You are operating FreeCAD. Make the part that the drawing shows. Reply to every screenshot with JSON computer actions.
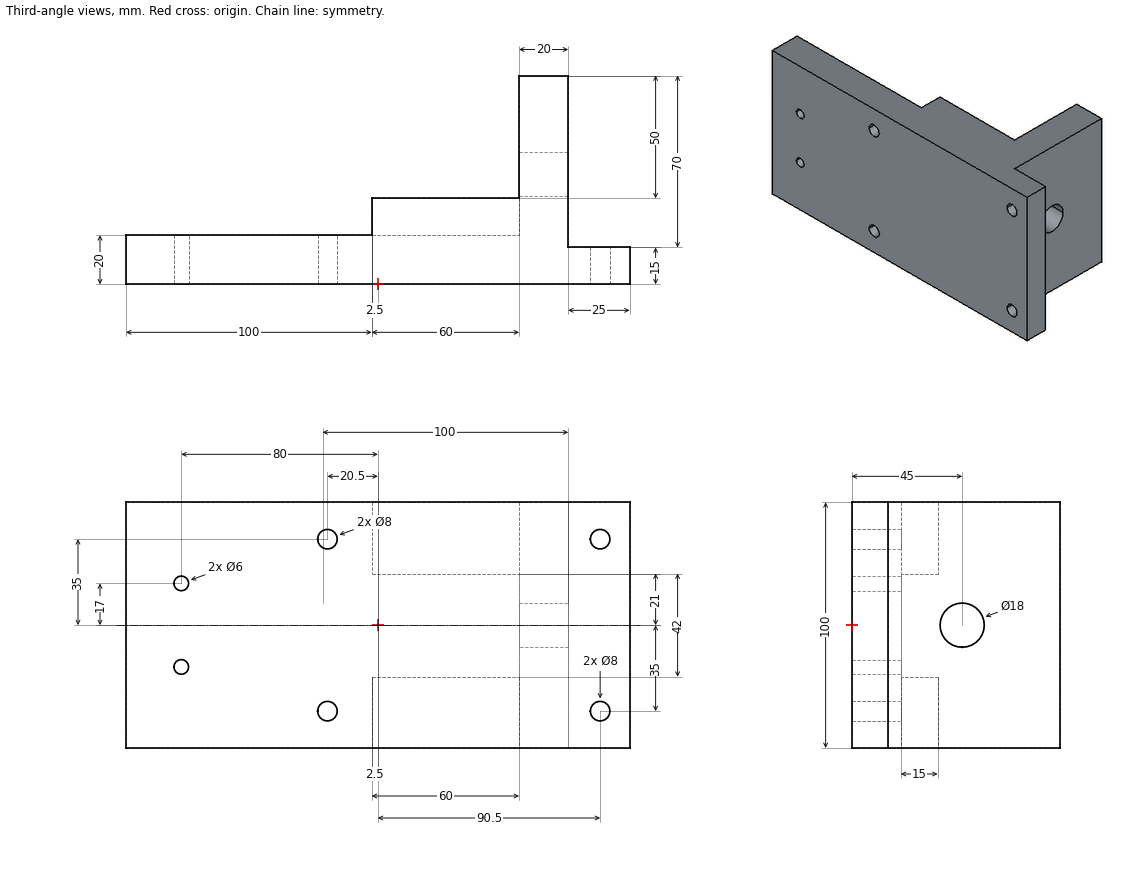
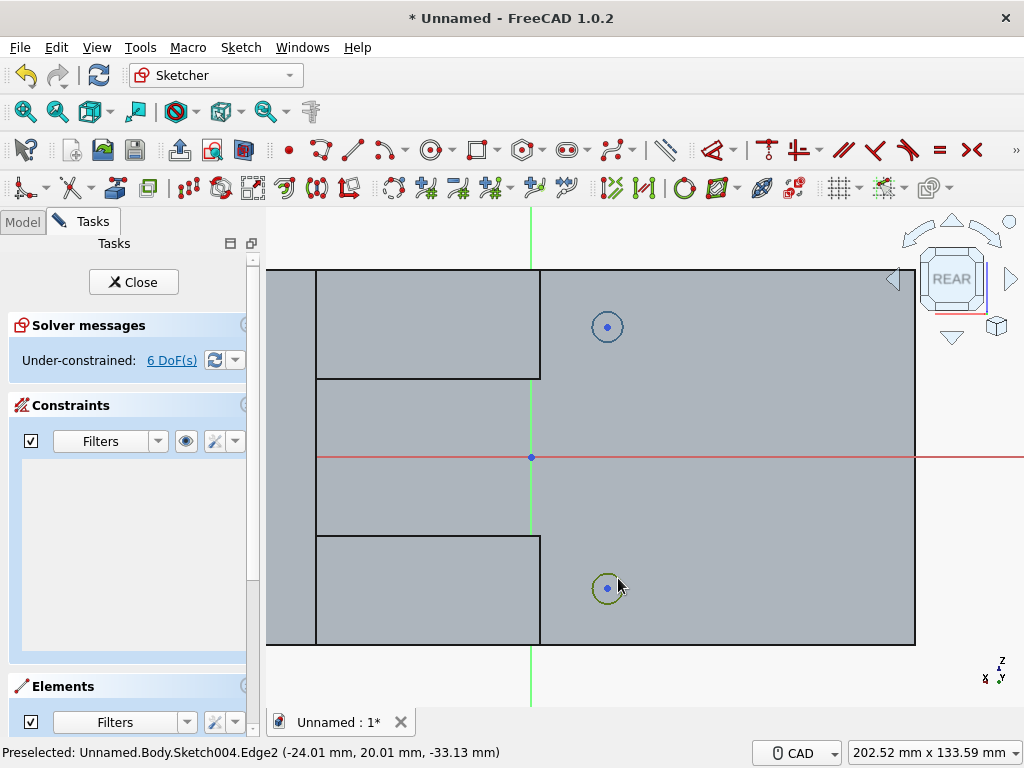
{"action": "left_click", "coordinate": [940, 150]}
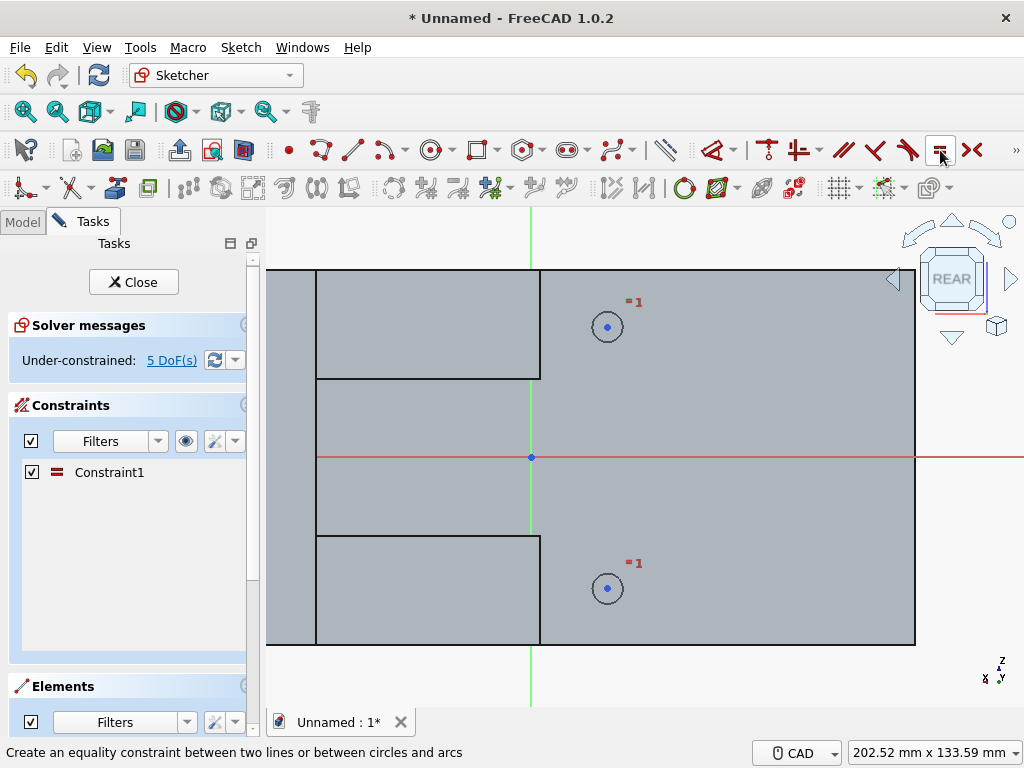
{"action": "left_click", "coordinate": [608, 327]}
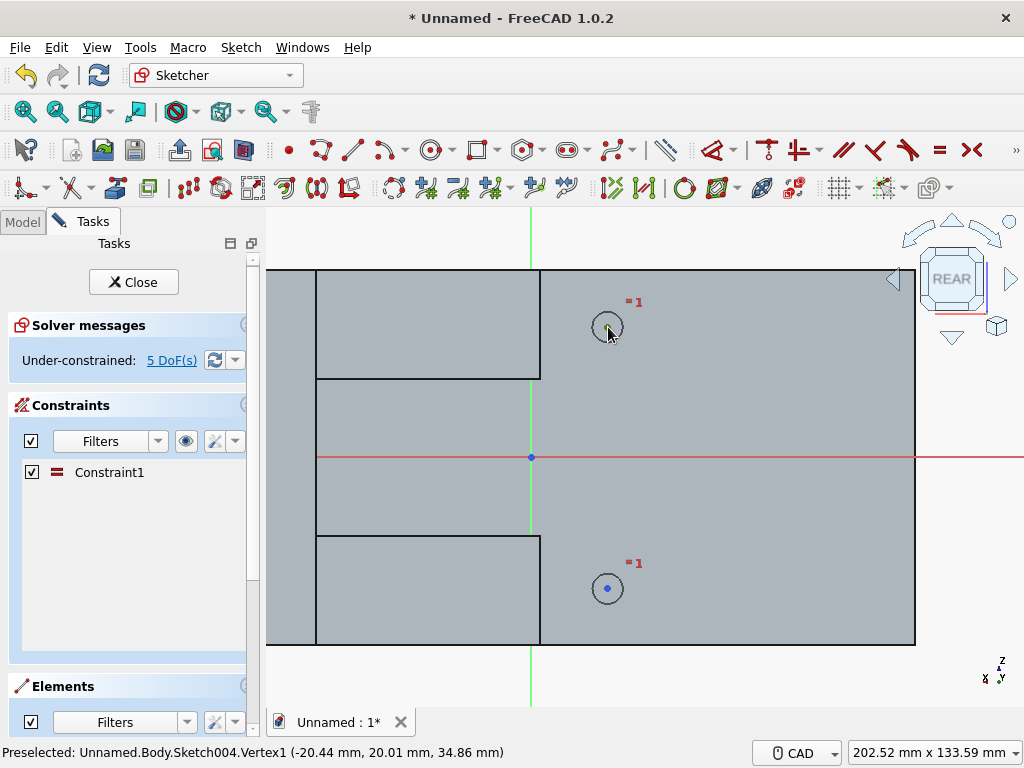
{"action": "left_click", "coordinate": [608, 589]}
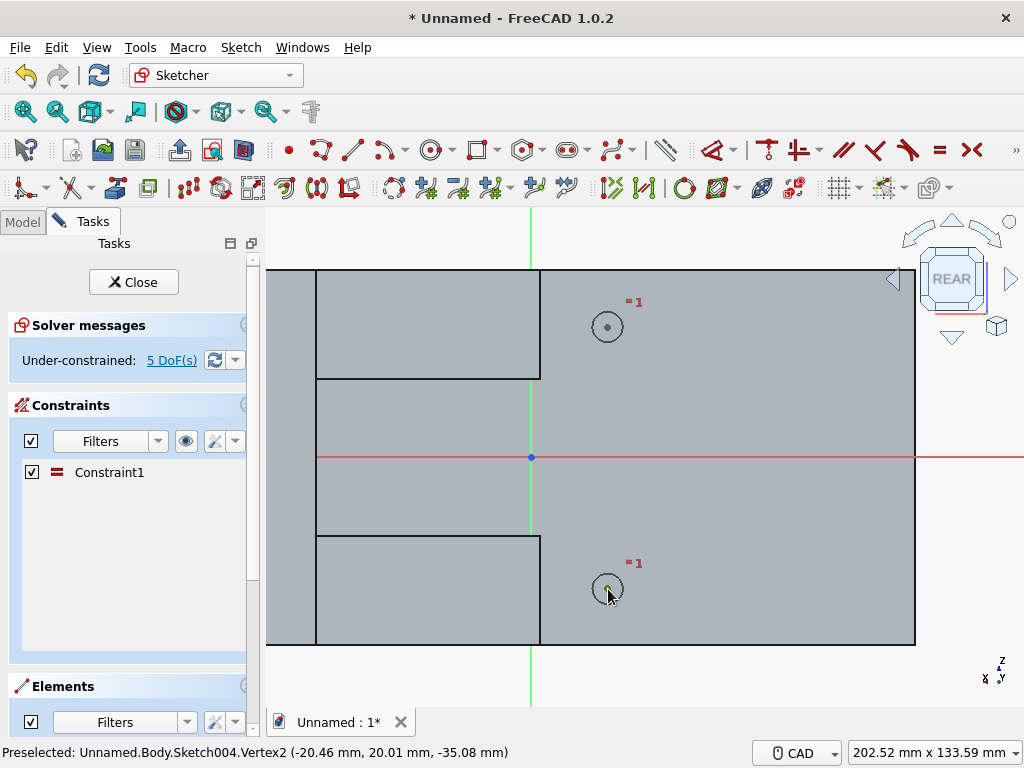
{"action": "left_click", "coordinate": [334, 457]}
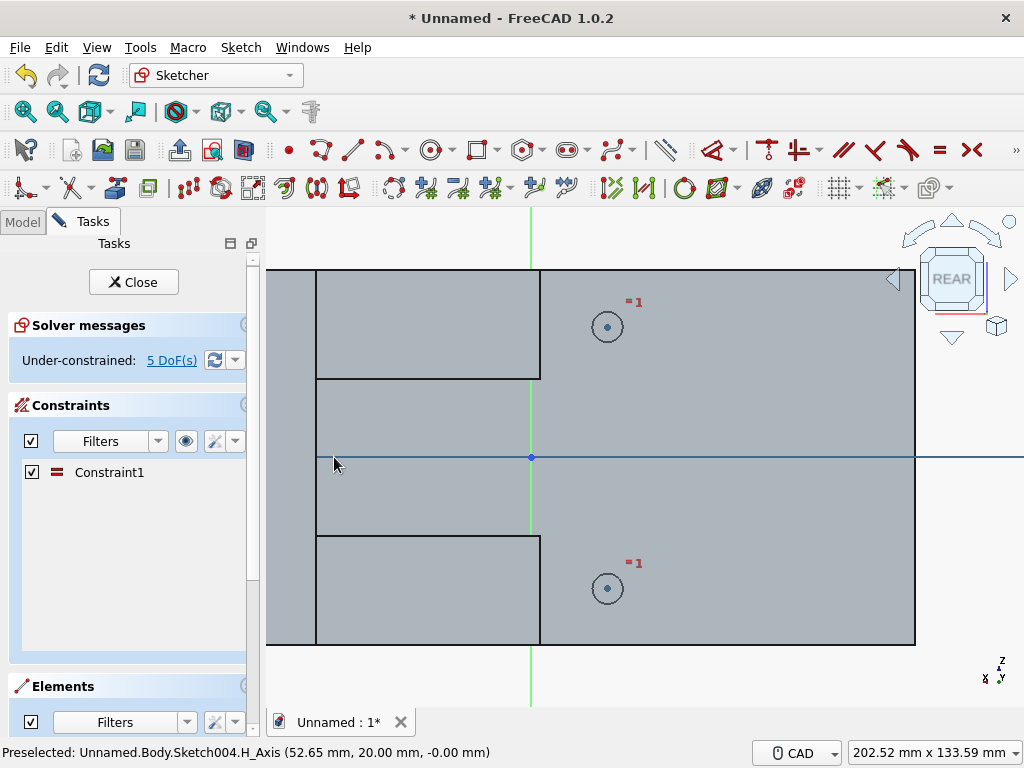
{"action": "left_click", "coordinate": [972, 150]}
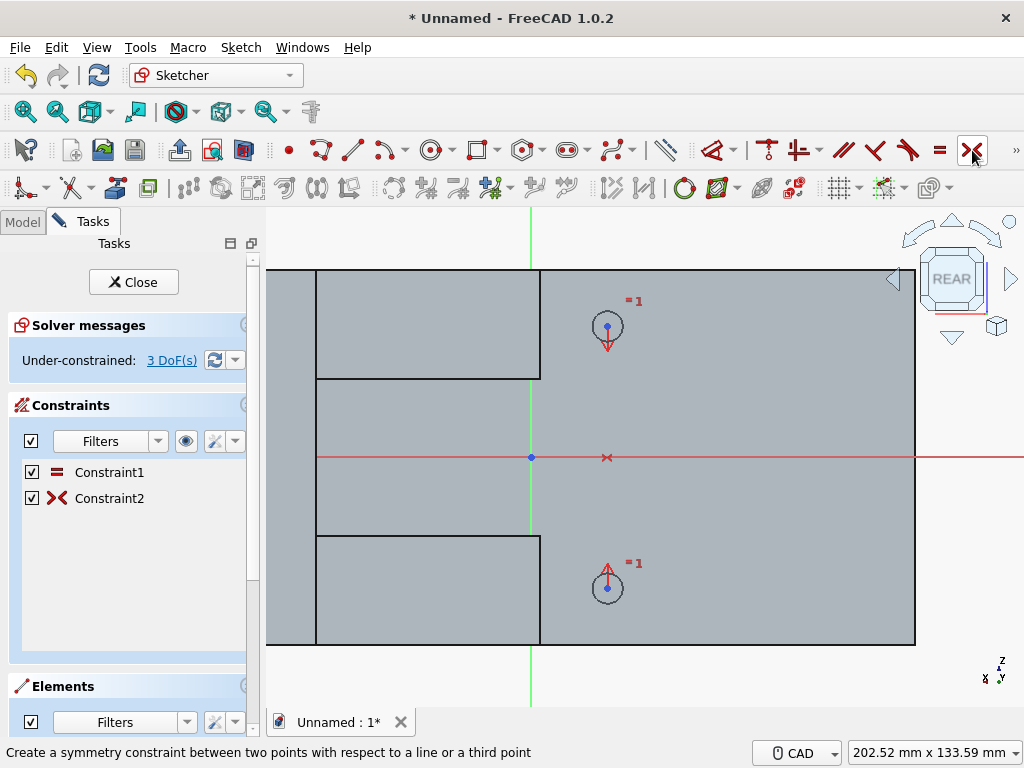
{"action": "left_click", "coordinate": [712, 150]}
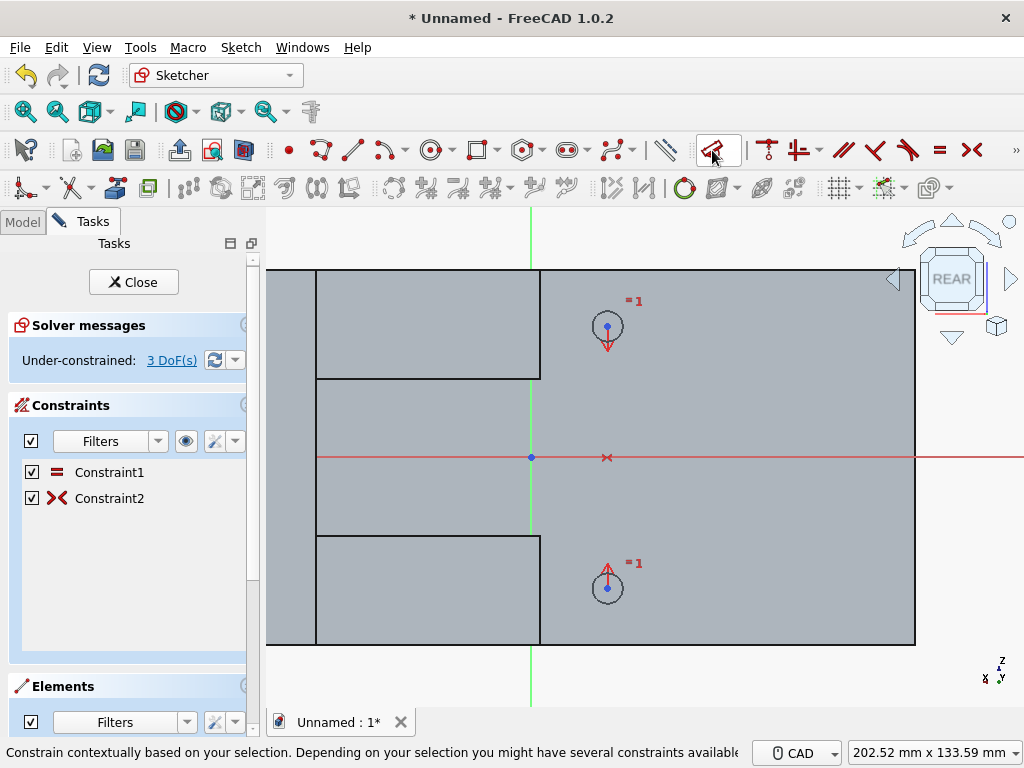
{"action": "scroll", "coordinate": [618, 316], "scroll_direction": "up", "scroll_amount": 2}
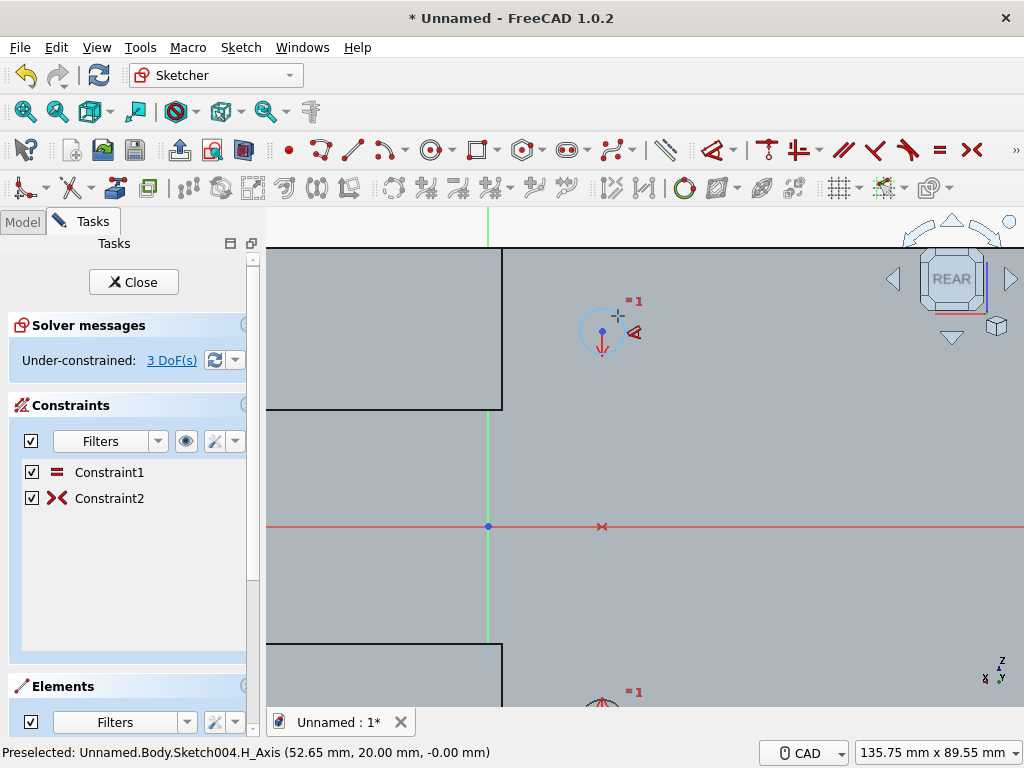
{"action": "left_click", "coordinate": [618, 315]}
{"action": "left_click", "coordinate": [640, 292]}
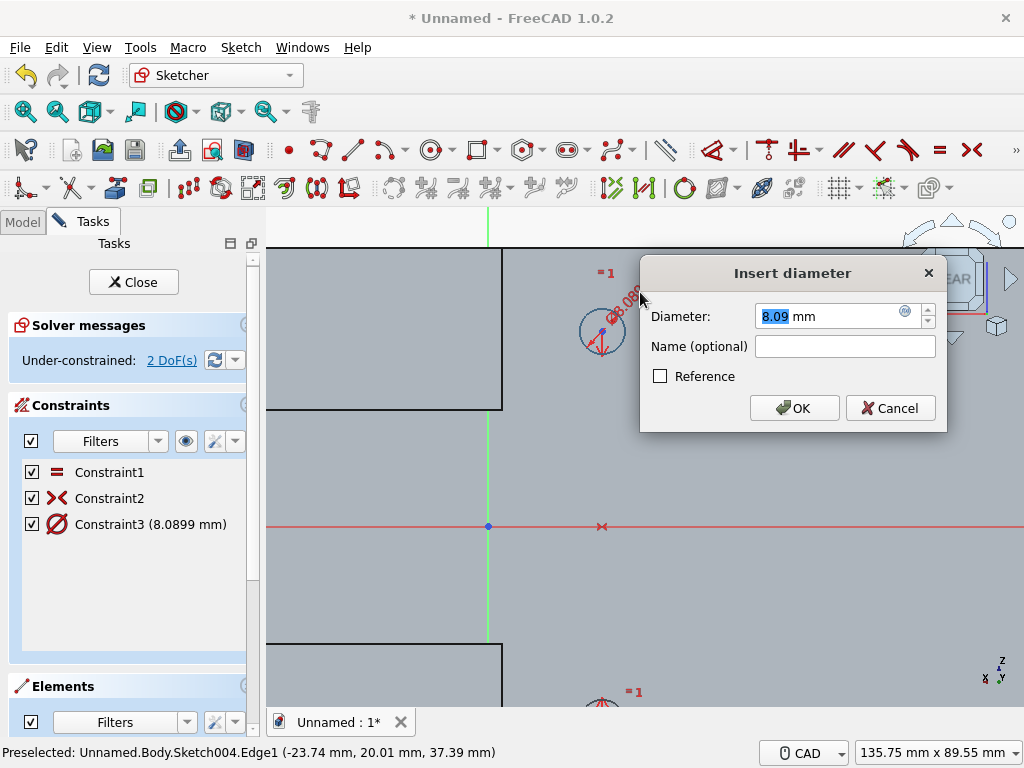
{"action": "type", "text": "8"}
{"action": "key", "text": "Return"}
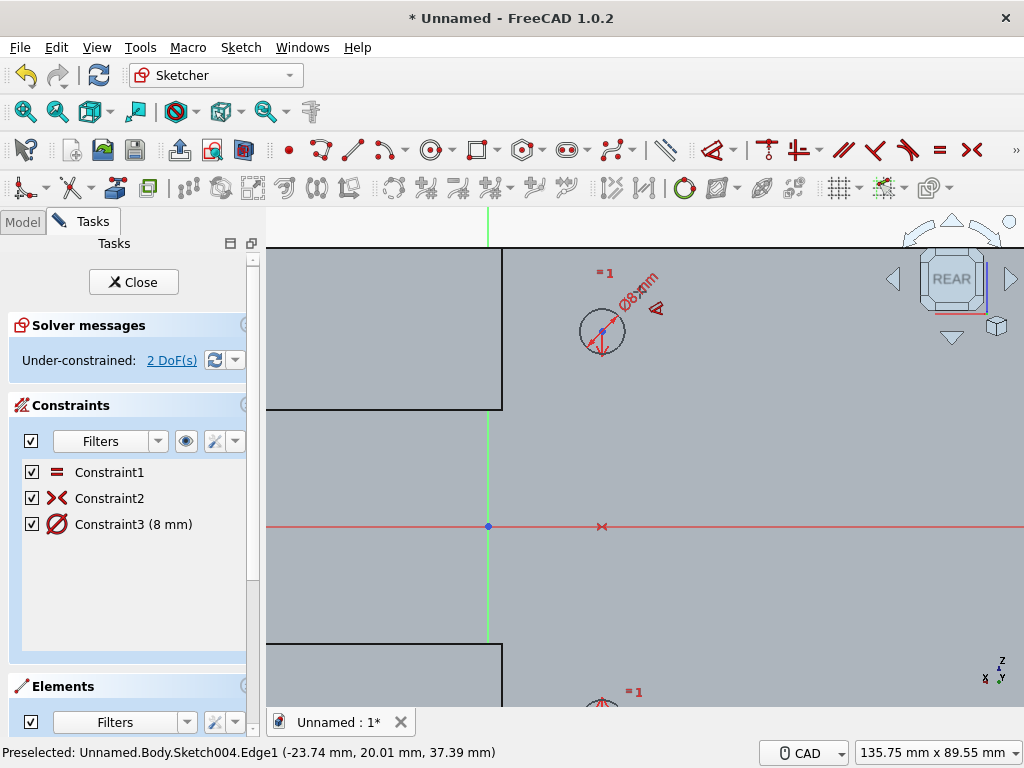
{"action": "left_click", "coordinate": [602, 331]}
{"action": "left_click", "coordinate": [454, 429]}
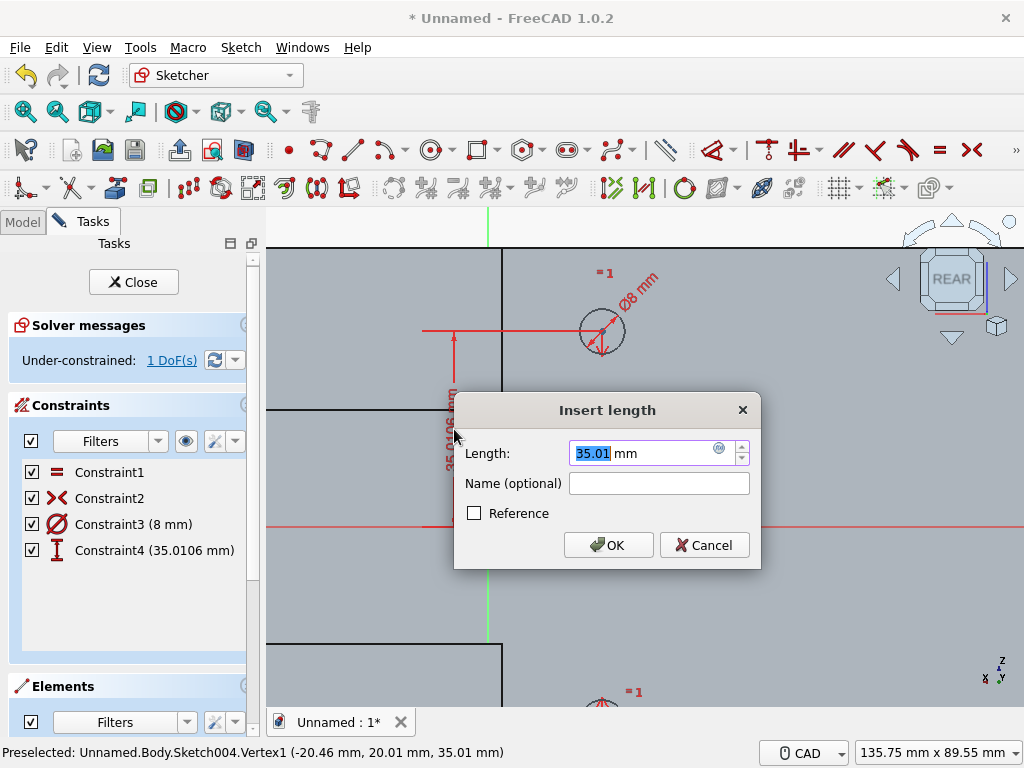
{"action": "type", "text": "35"}
{"action": "key", "text": "Return"}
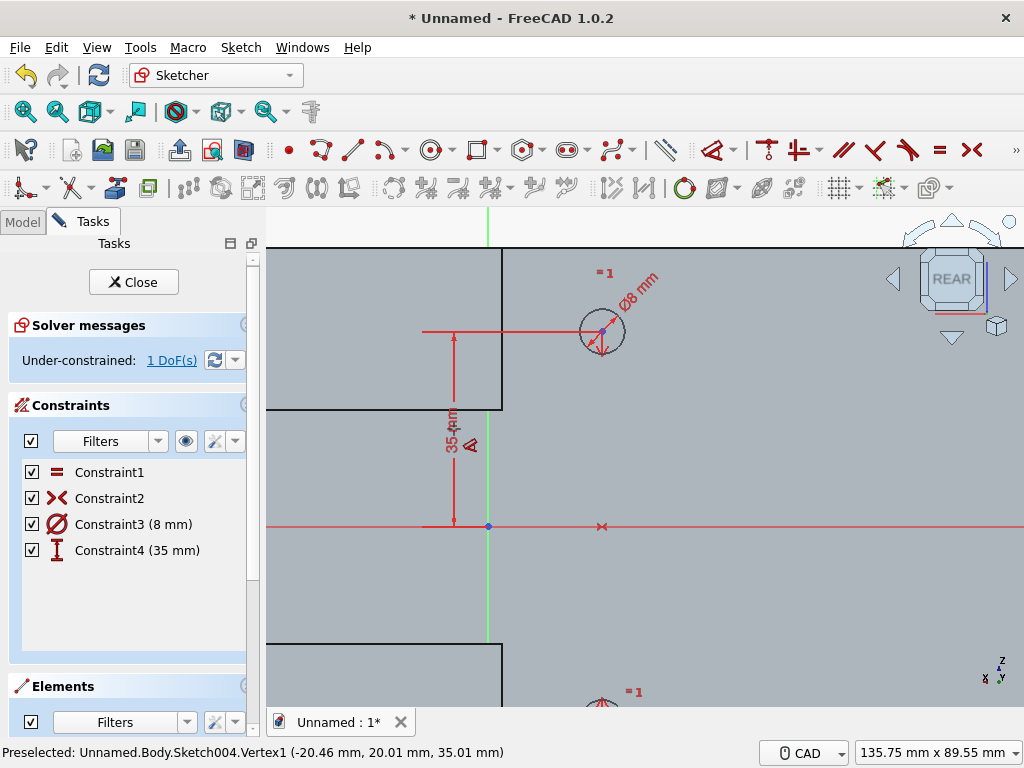
{"action": "left_click", "coordinate": [602, 332]}
{"action": "left_click", "coordinate": [545, 298]}